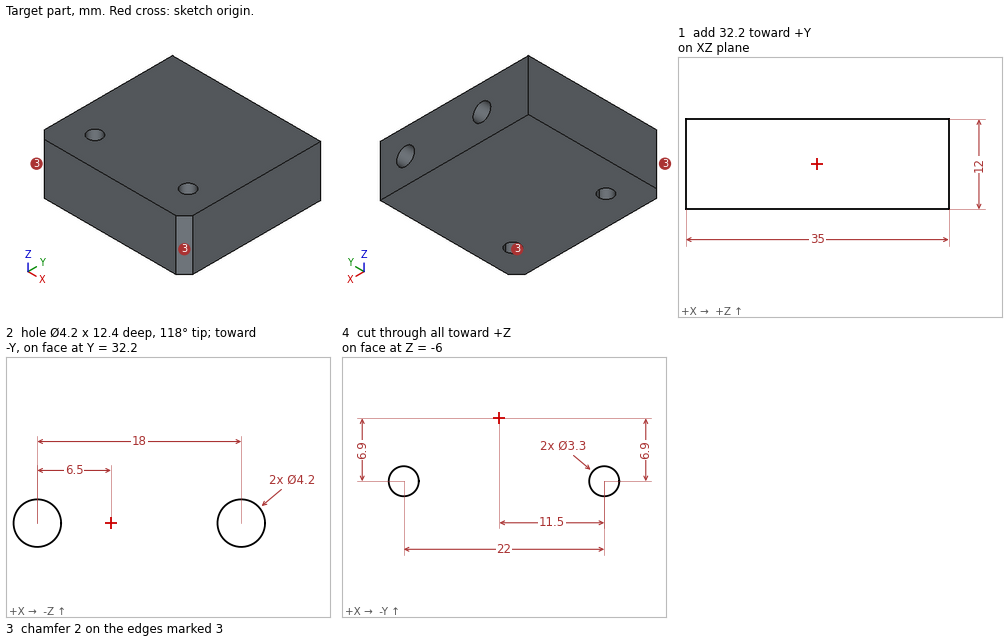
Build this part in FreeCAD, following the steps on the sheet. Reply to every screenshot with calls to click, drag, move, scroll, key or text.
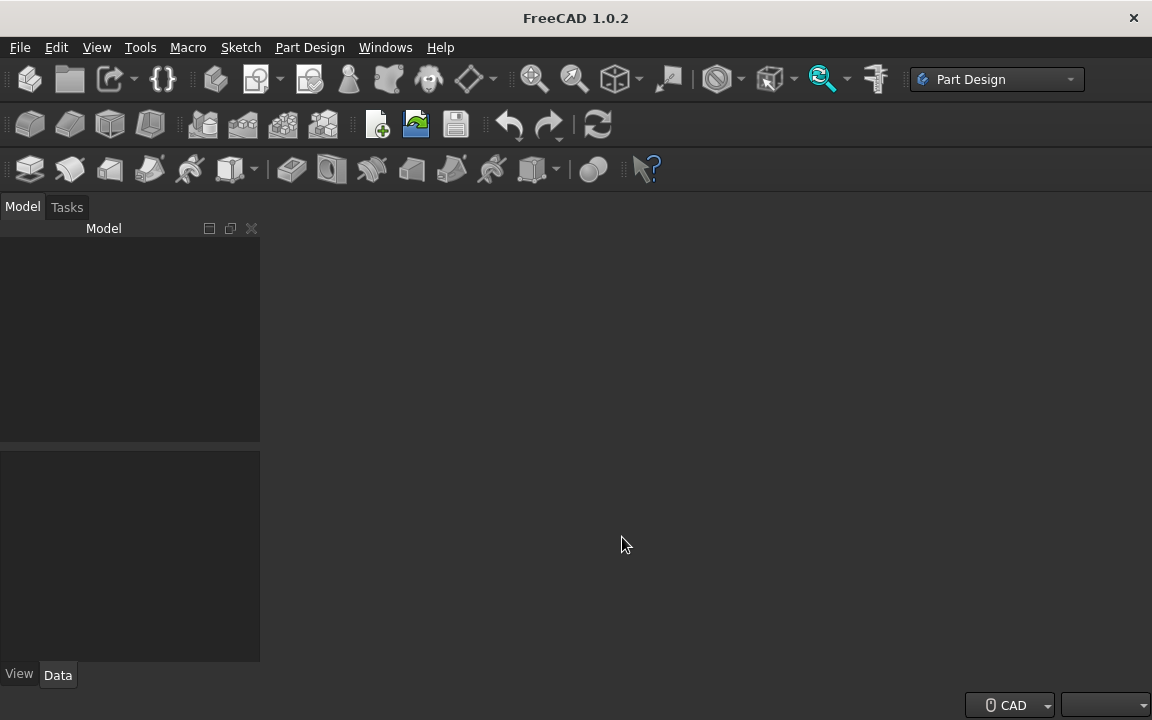
key(ctrl+n)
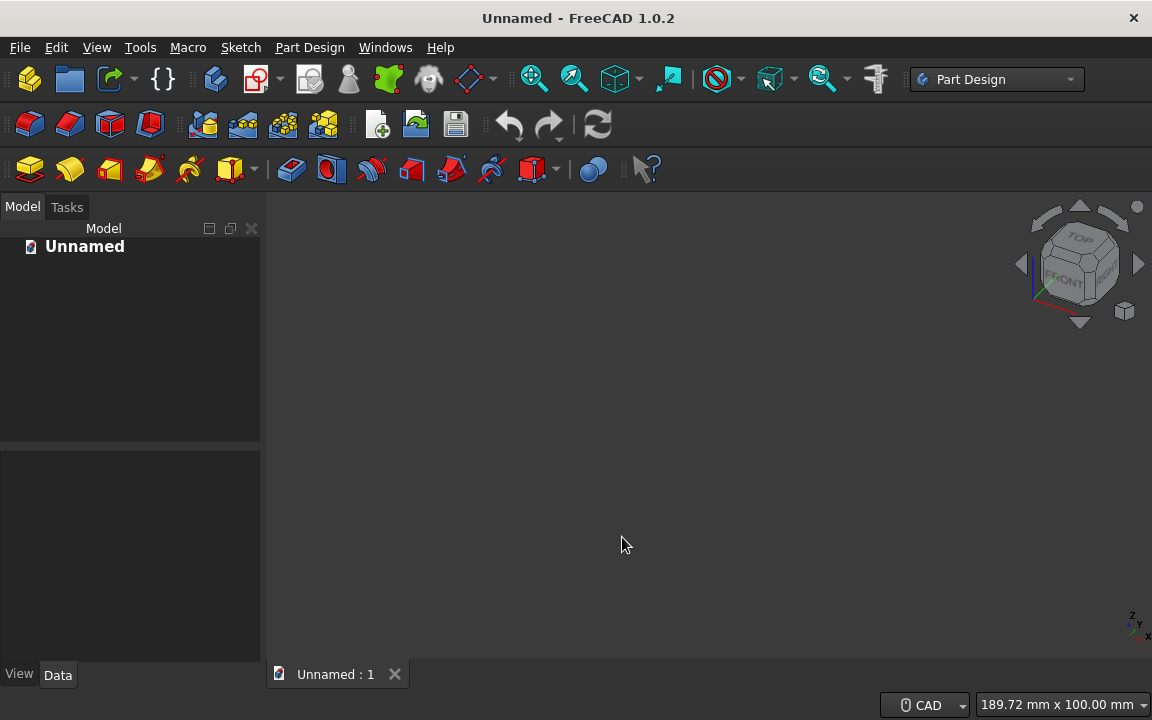
click(256, 80)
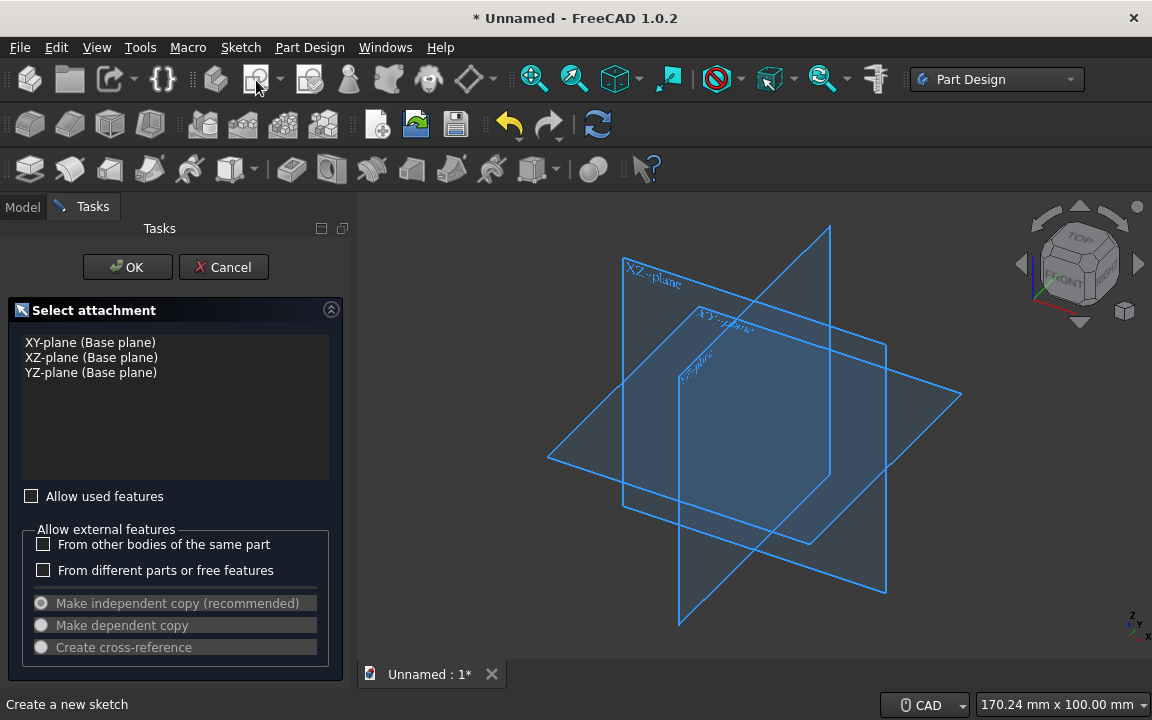
click(82, 358)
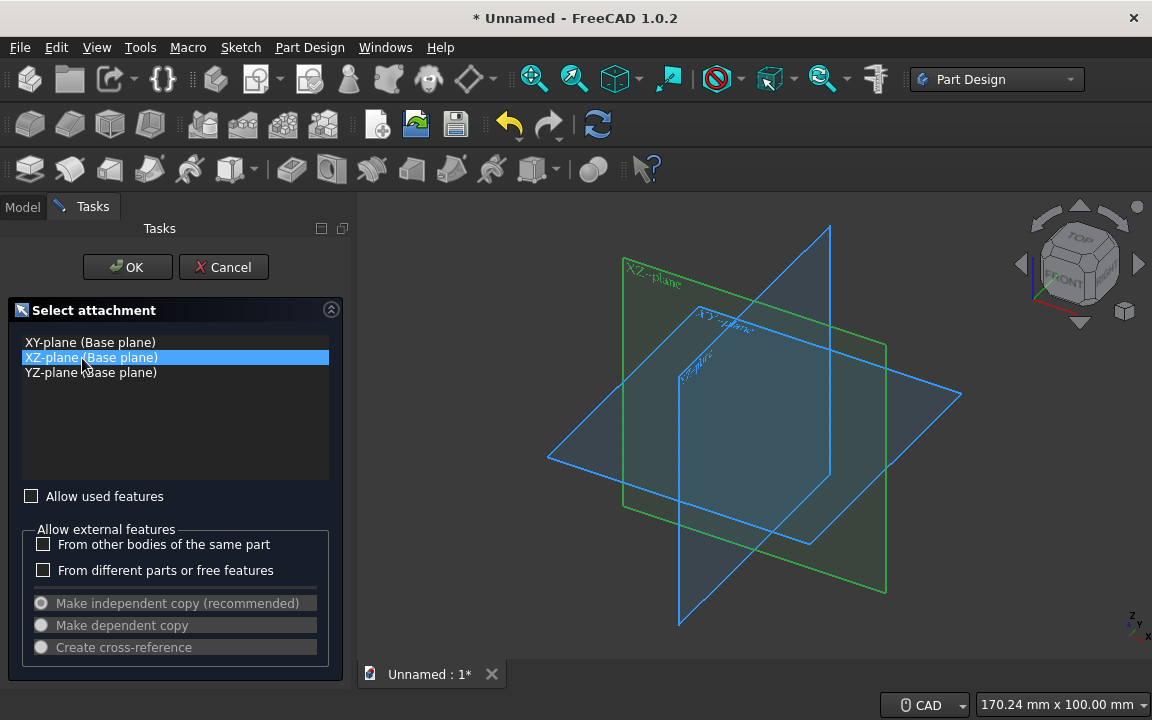
click(128, 267)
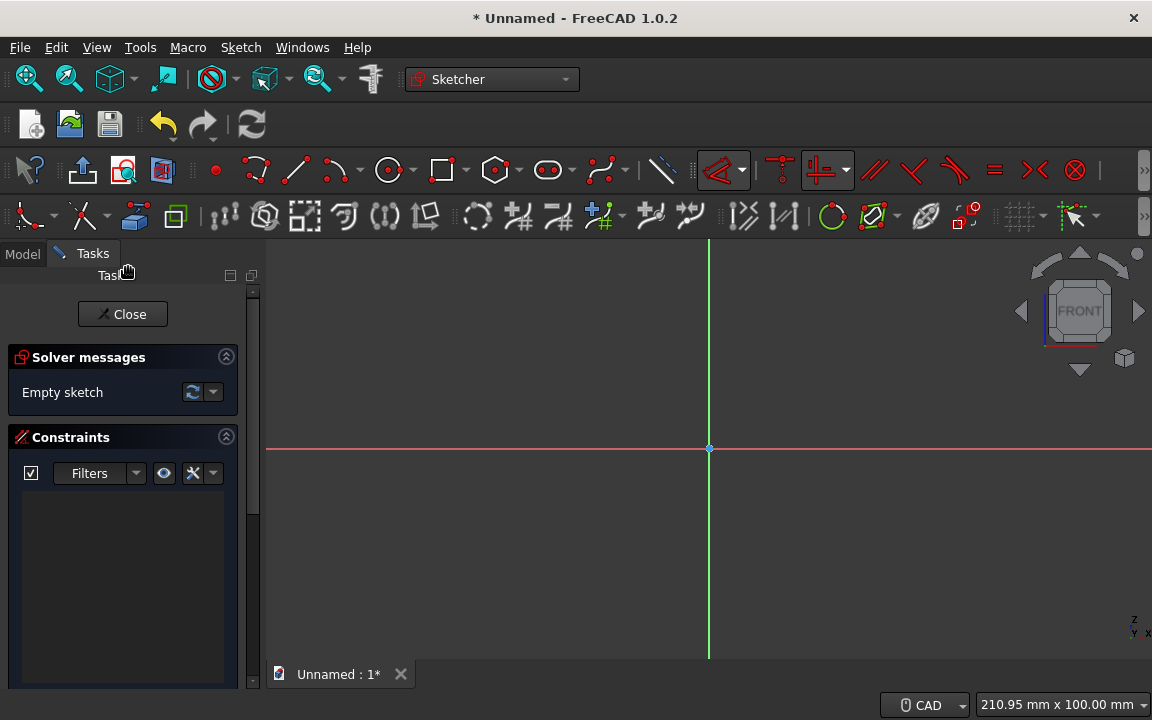
scroll(739, 449, up, 6)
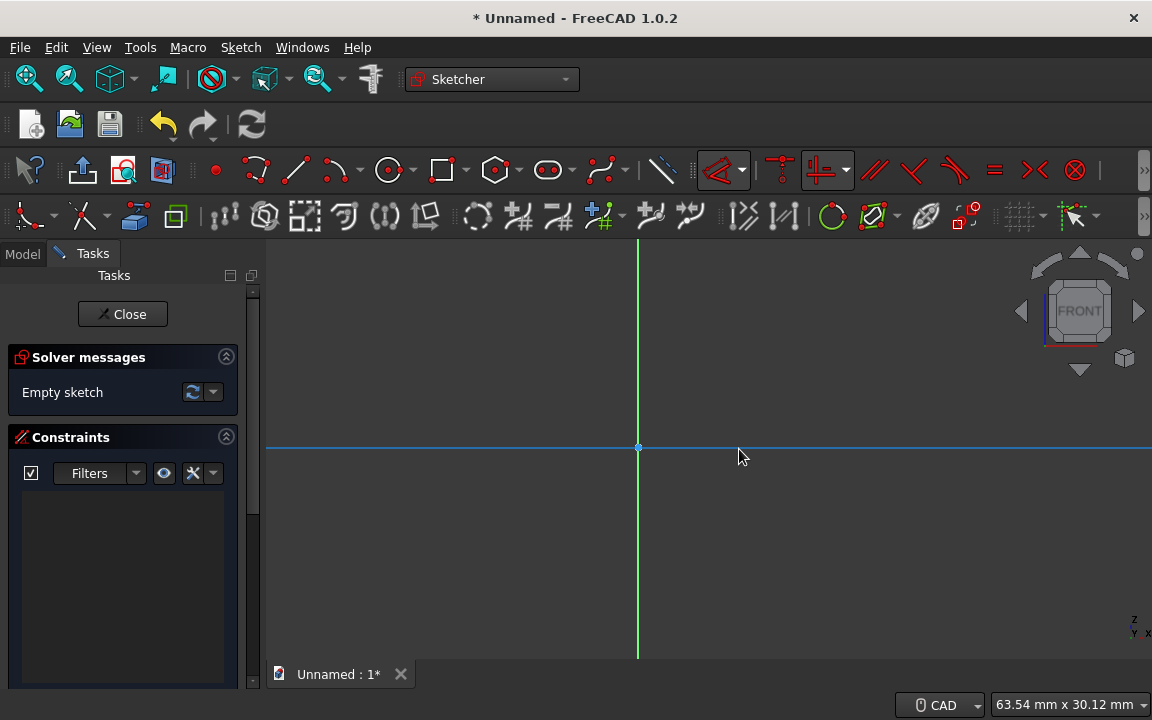
key(g)
key(v)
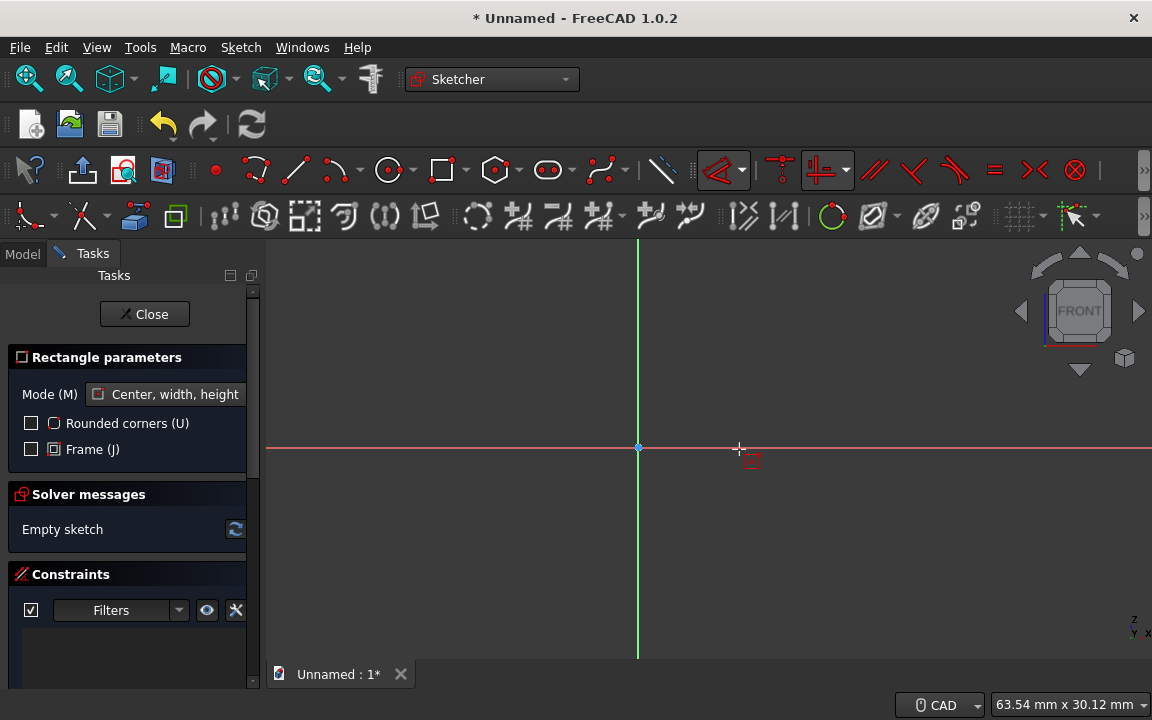
click(638, 448)
move(882, 364)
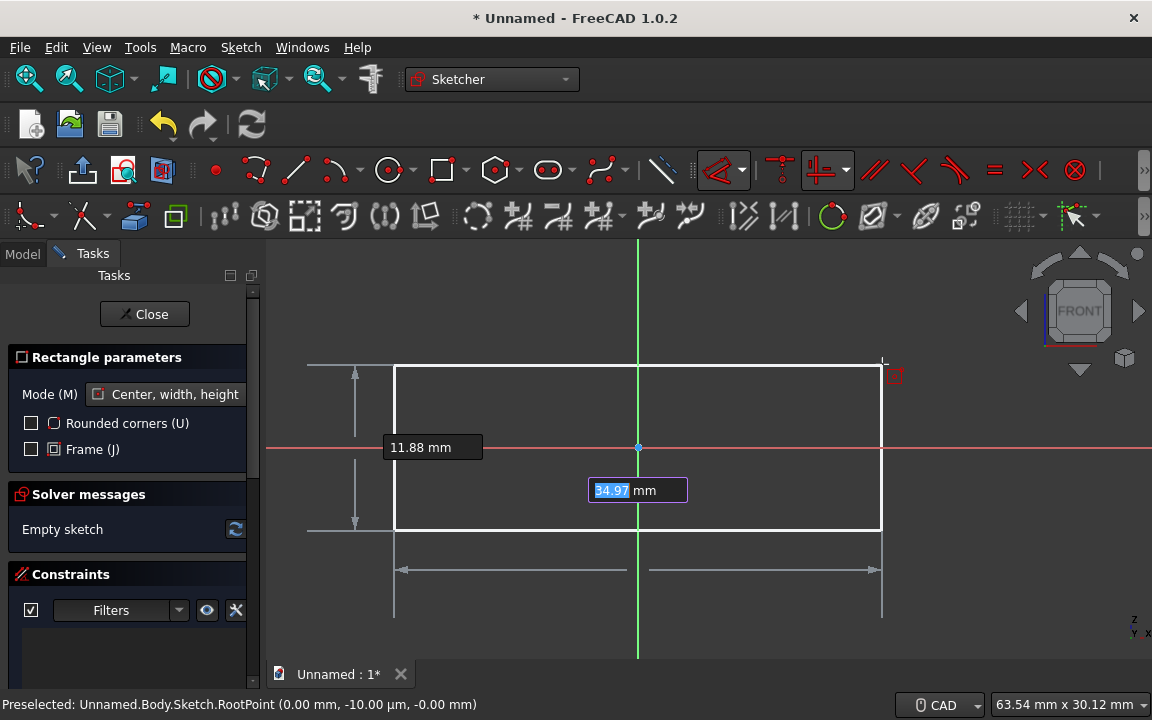
text(35)
key(Tab)
text(12)
key(Return)
key(Escape)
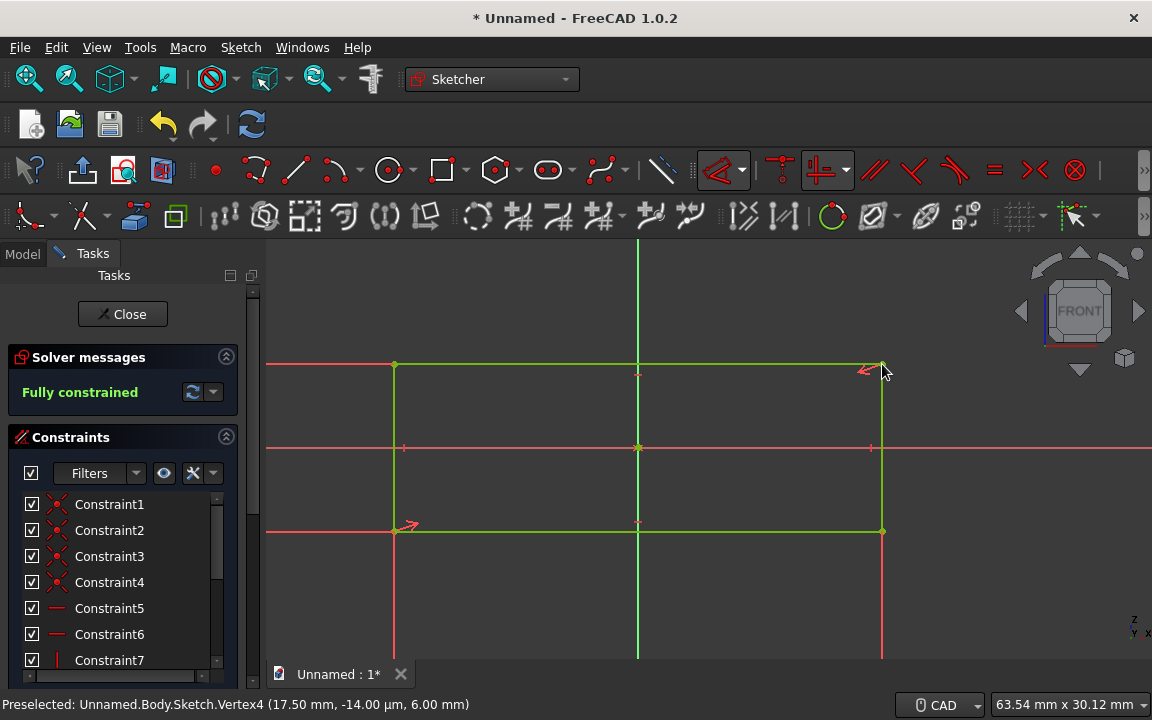
click(123, 314)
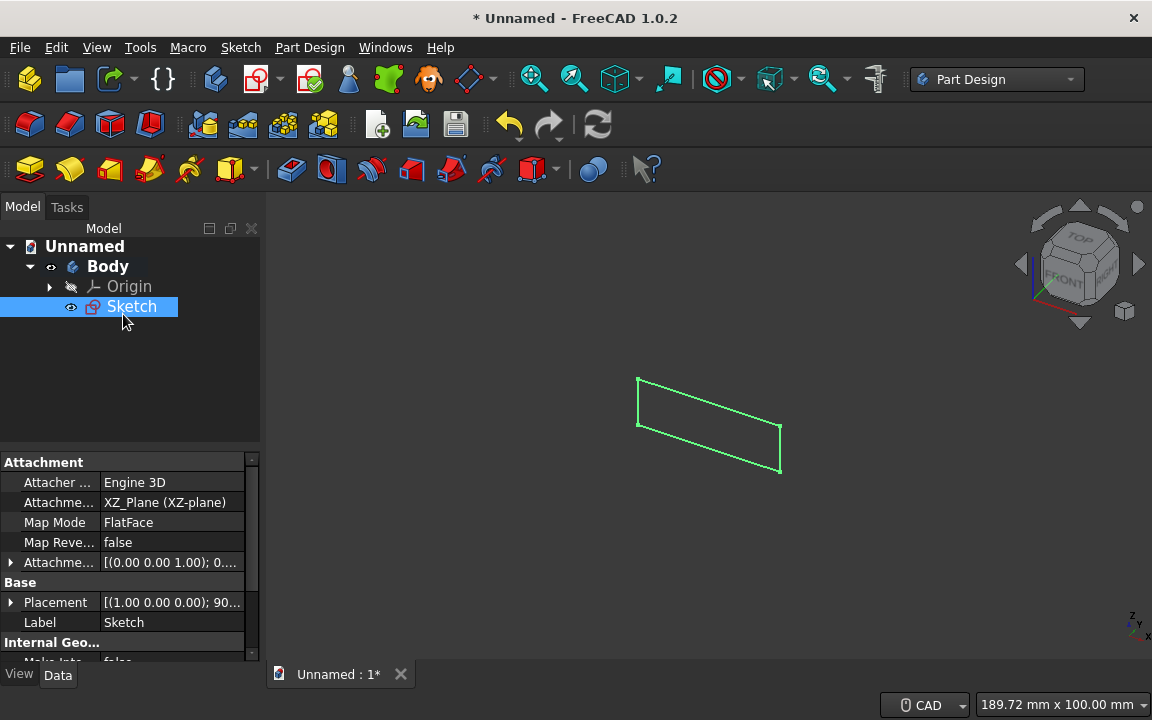
click(30, 170)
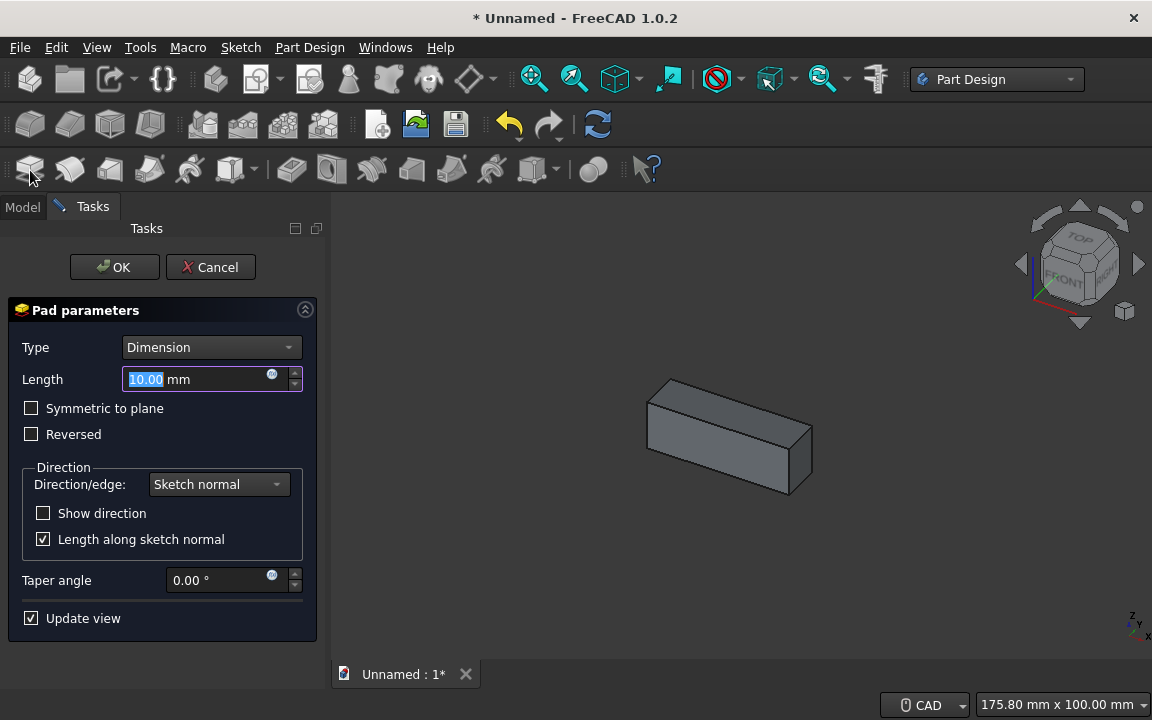
text(32.2)
key(Tab)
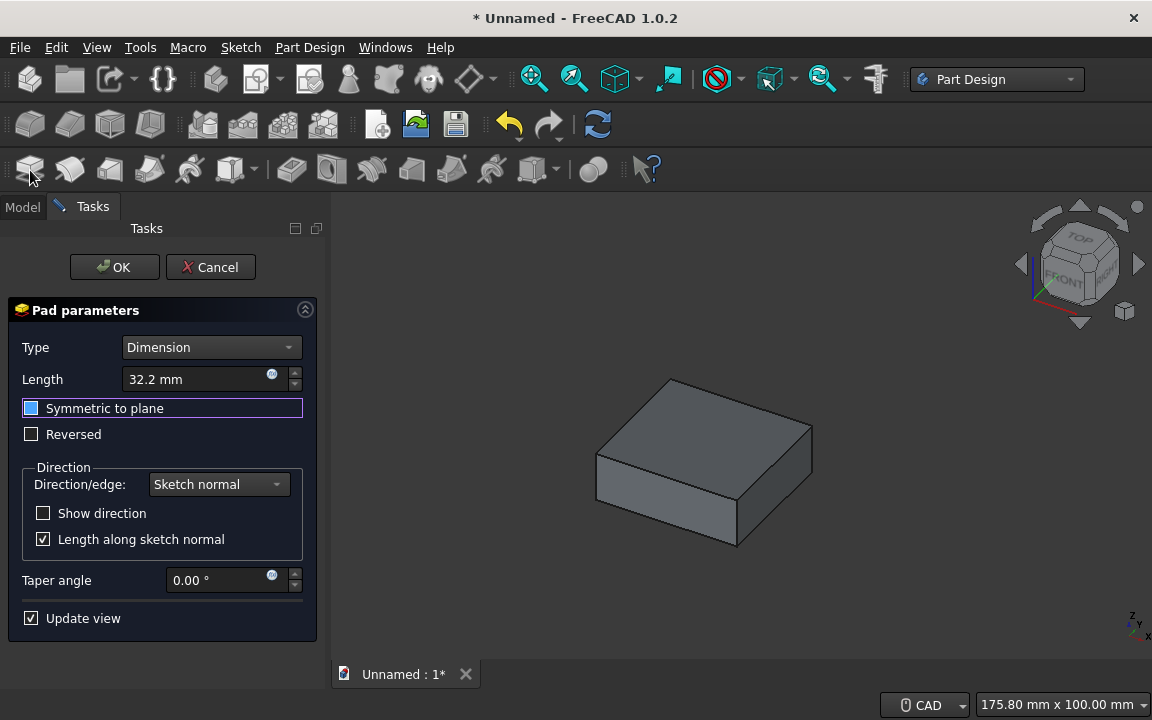
click(30, 434)